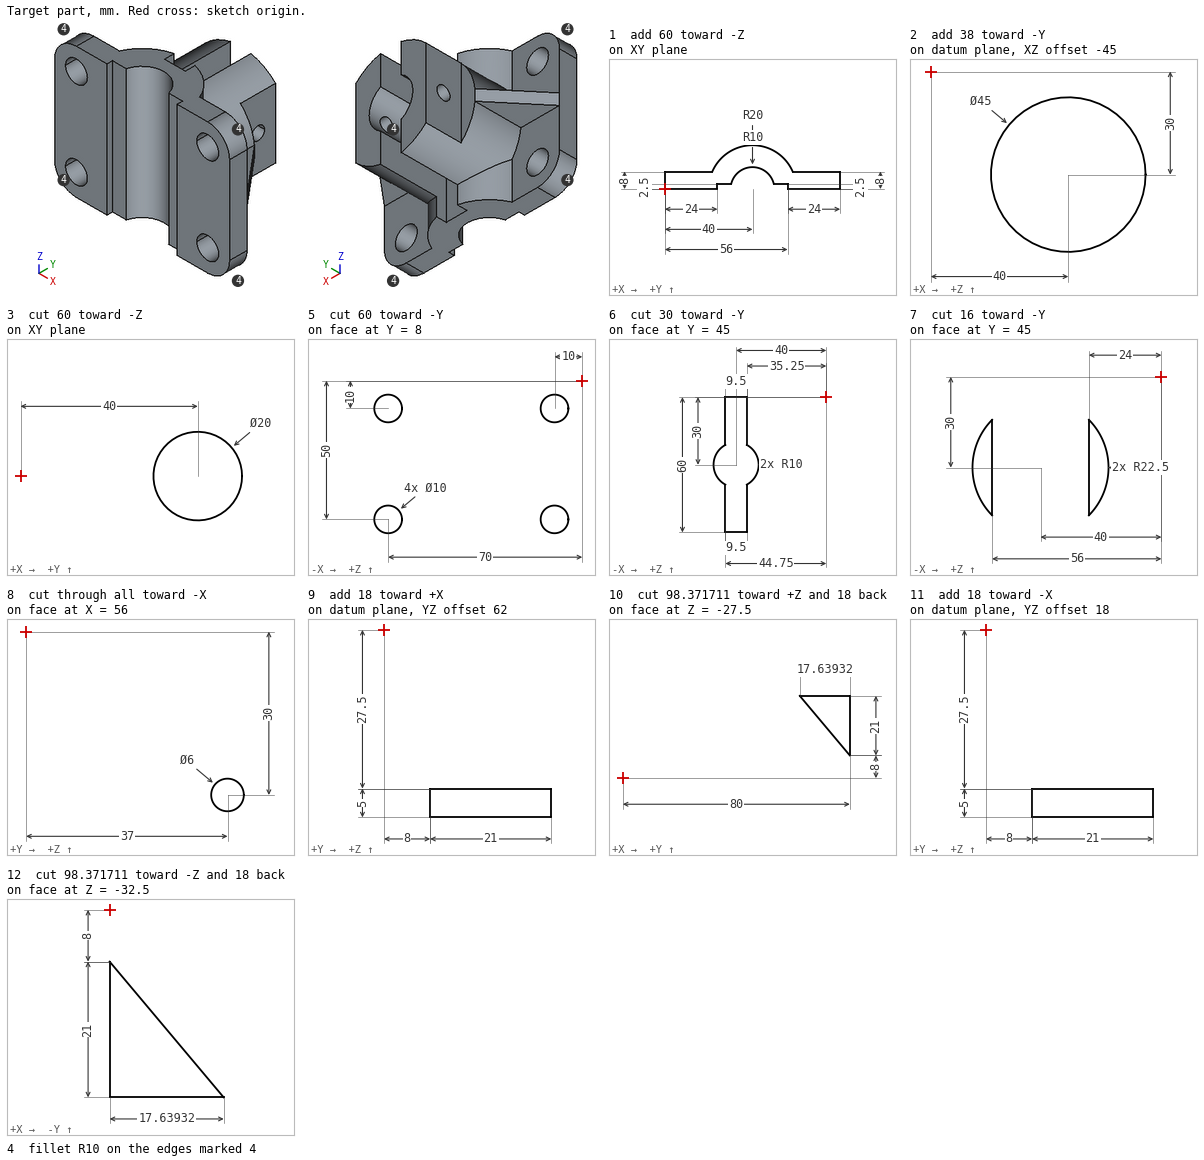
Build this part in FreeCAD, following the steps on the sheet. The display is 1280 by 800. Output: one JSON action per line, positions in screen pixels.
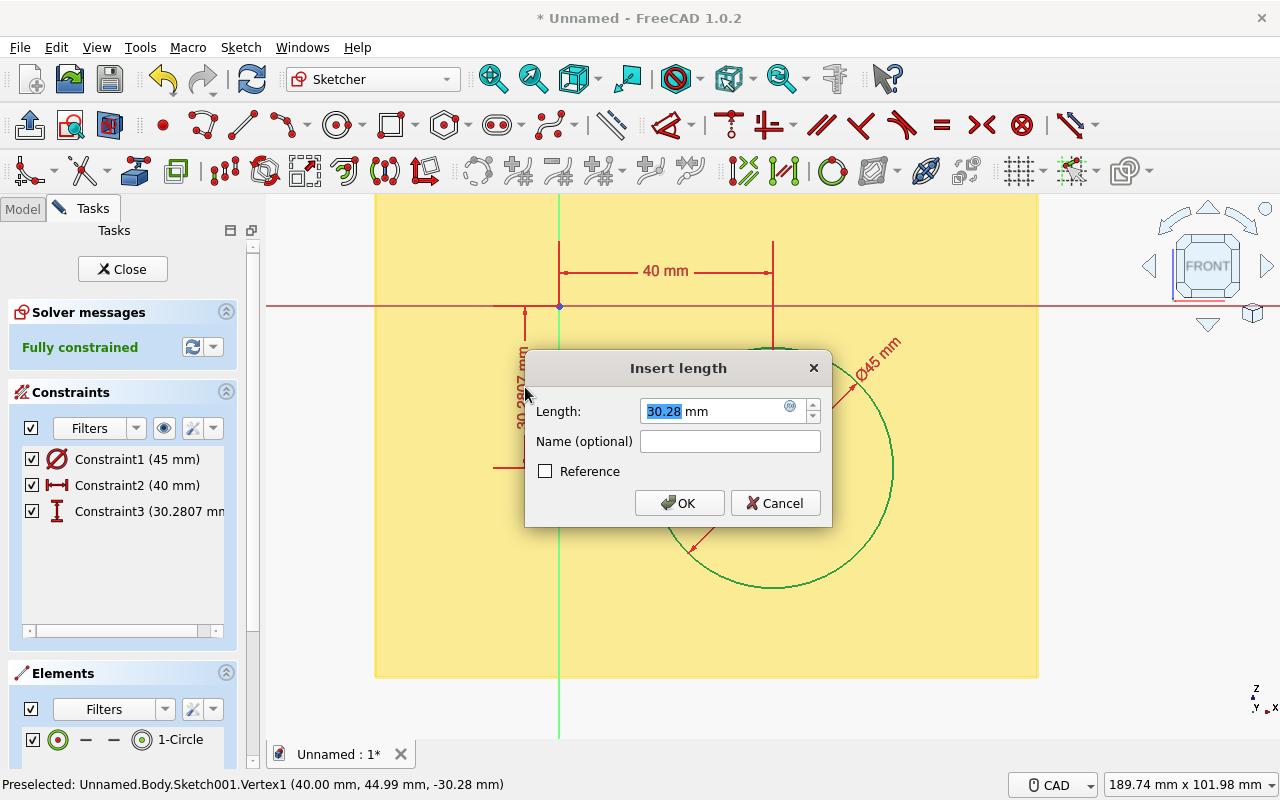
{"action": "type", "text": "30"}
{"action": "key", "text": "Return"}
{"action": "key", "text": "Escape"}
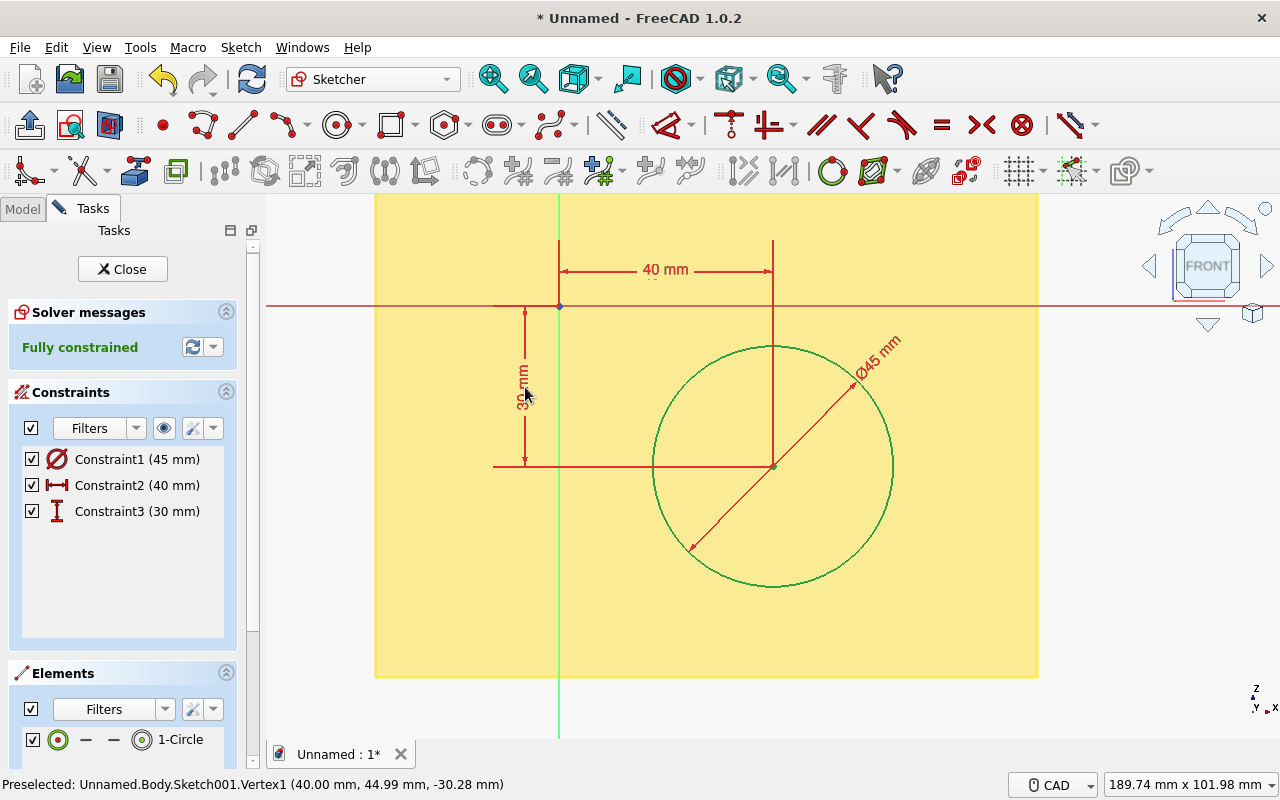
{"action": "left_click", "coordinate": [123, 269]}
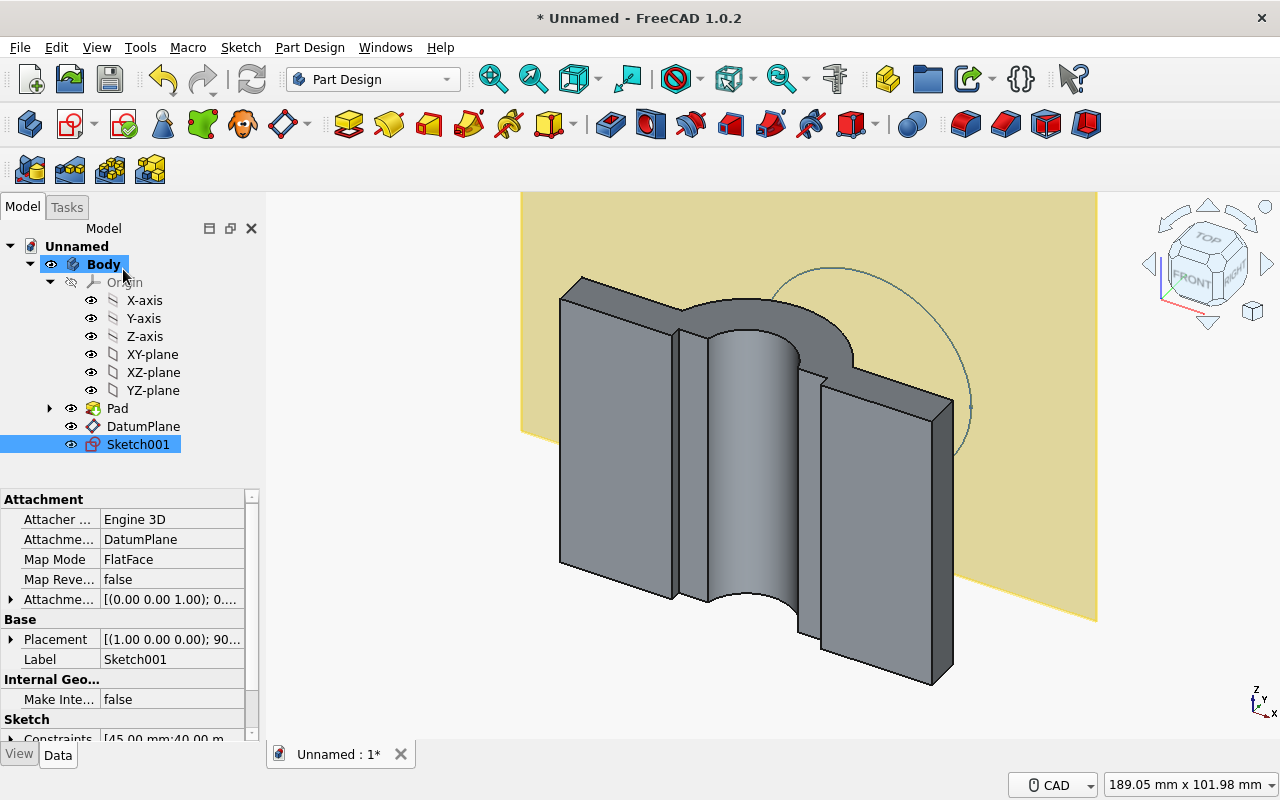
{"action": "left_click", "coordinate": [350, 124]}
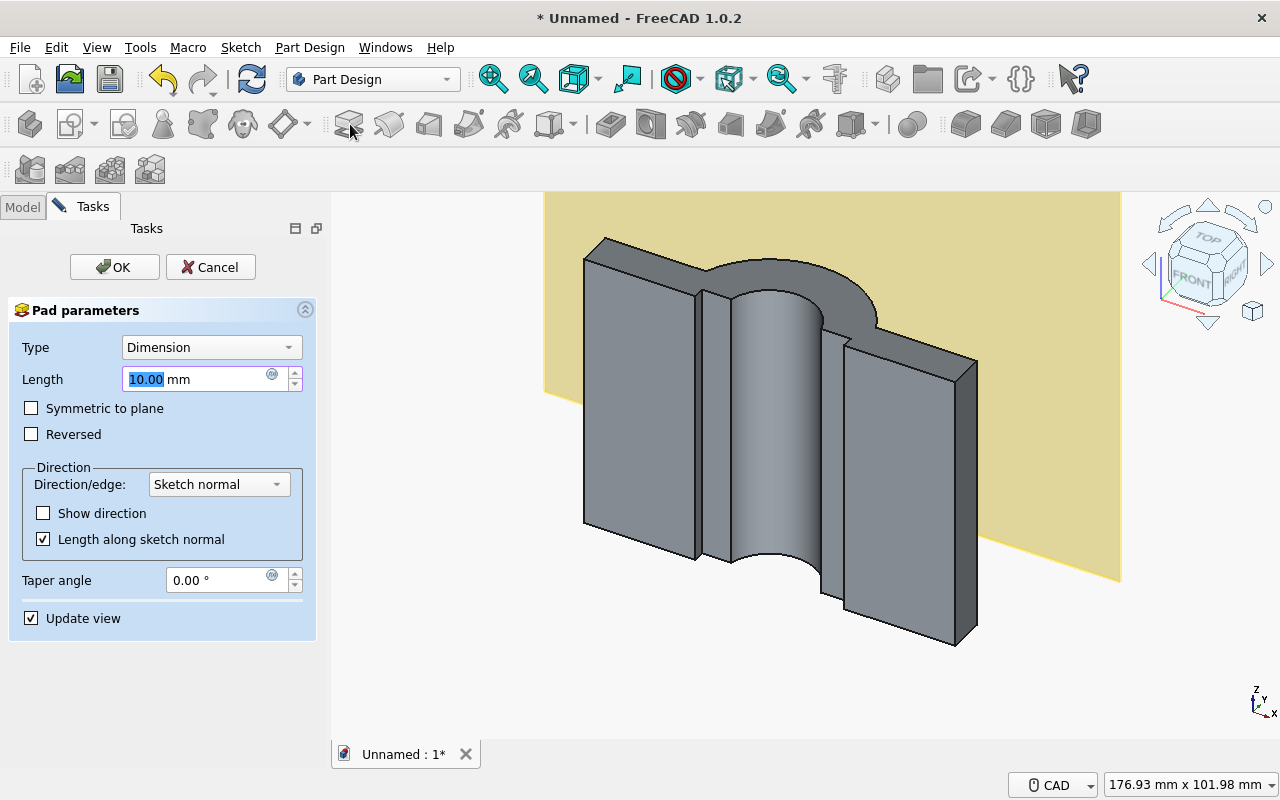
{"action": "type", "text": "38"}
{"action": "key", "text": "Tab"}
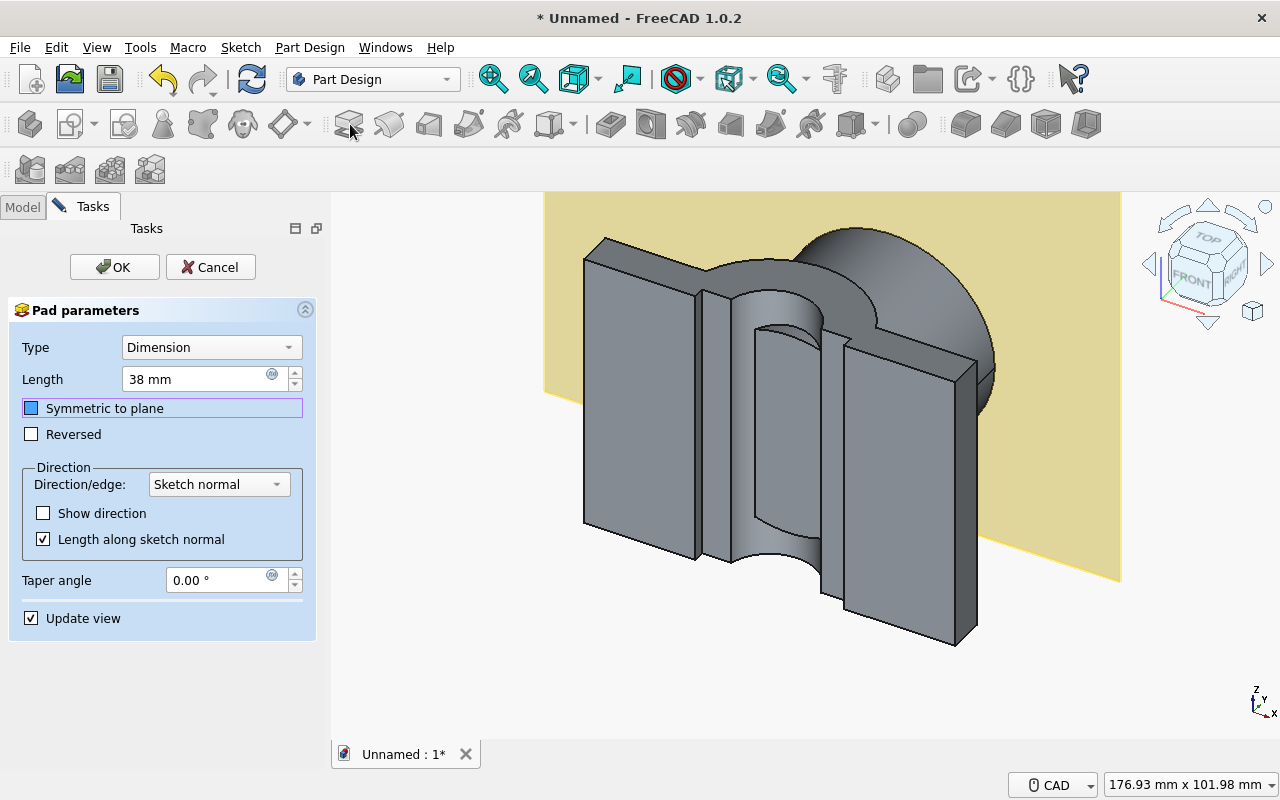
{"action": "left_click", "coordinate": [115, 267]}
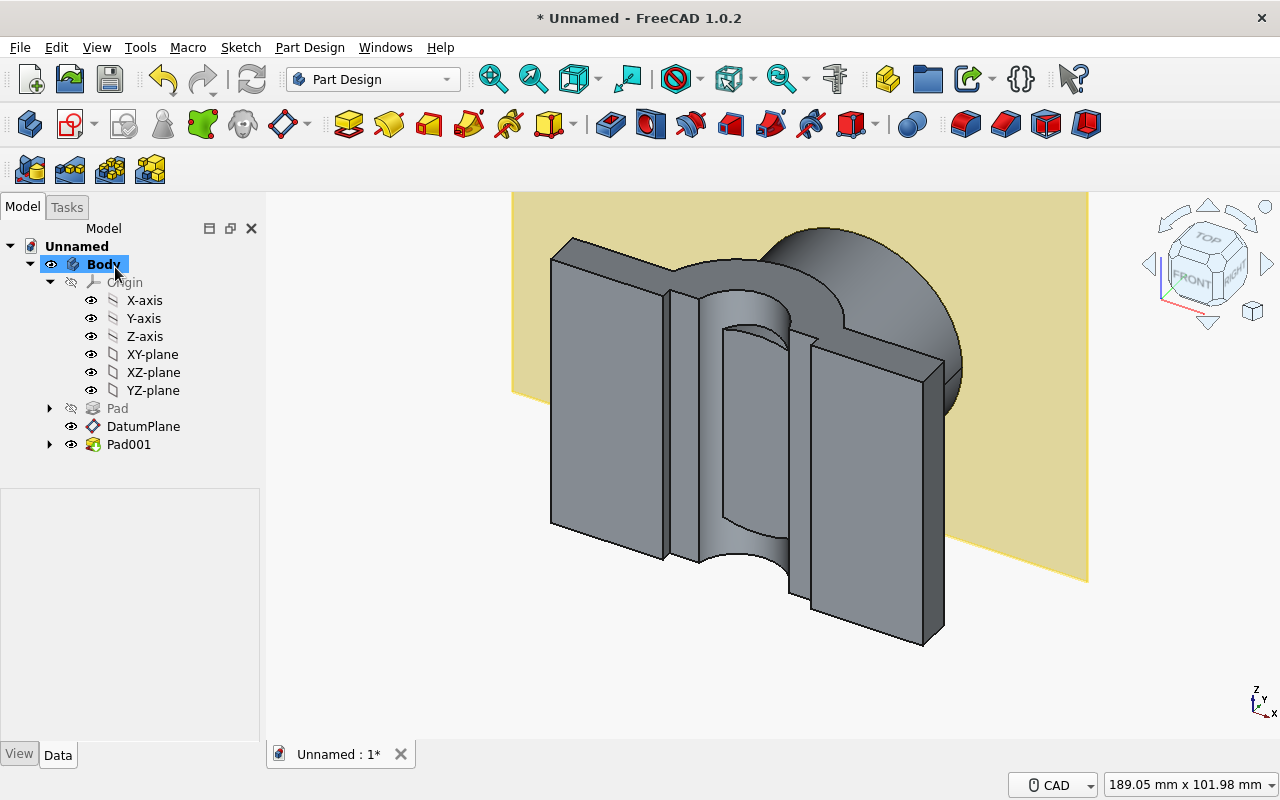
{"action": "left_click", "coordinate": [116, 426]}
{"action": "key", "text": "space"}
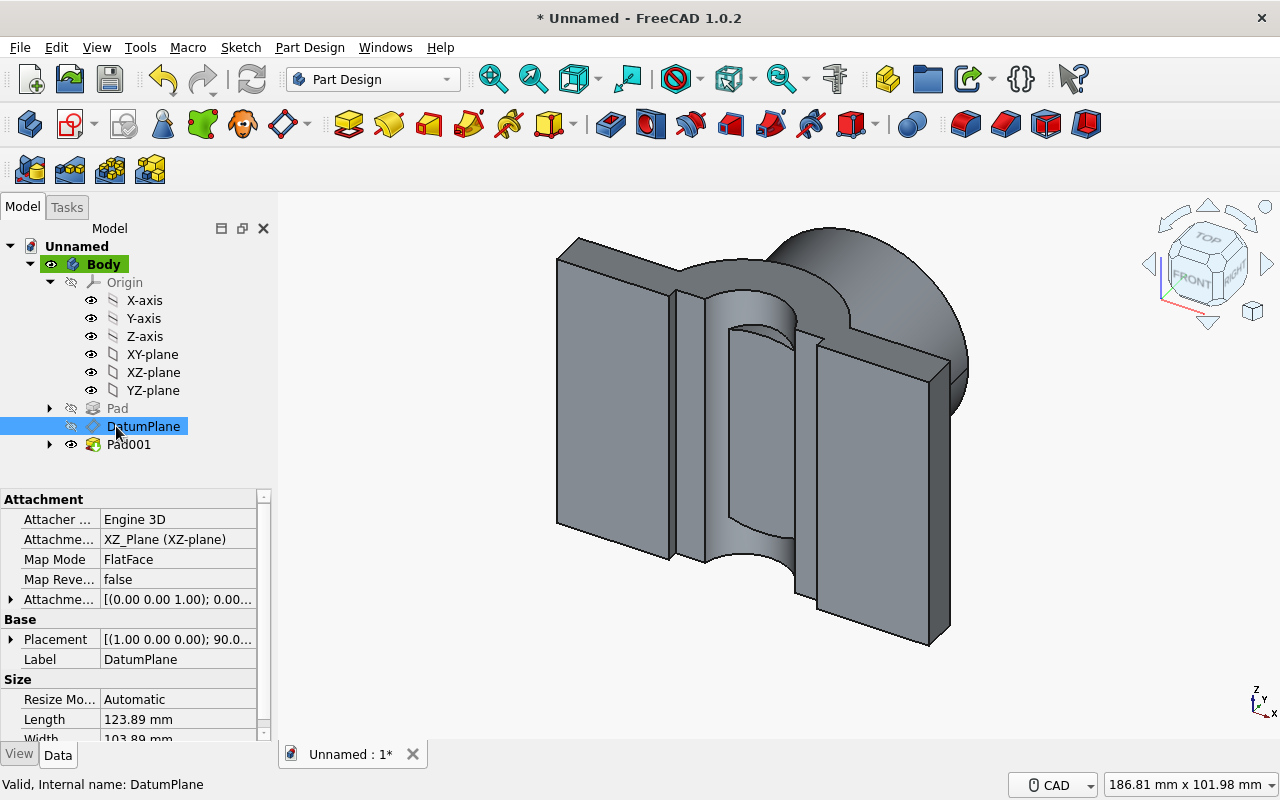
{"action": "left_click", "coordinate": [494, 80]}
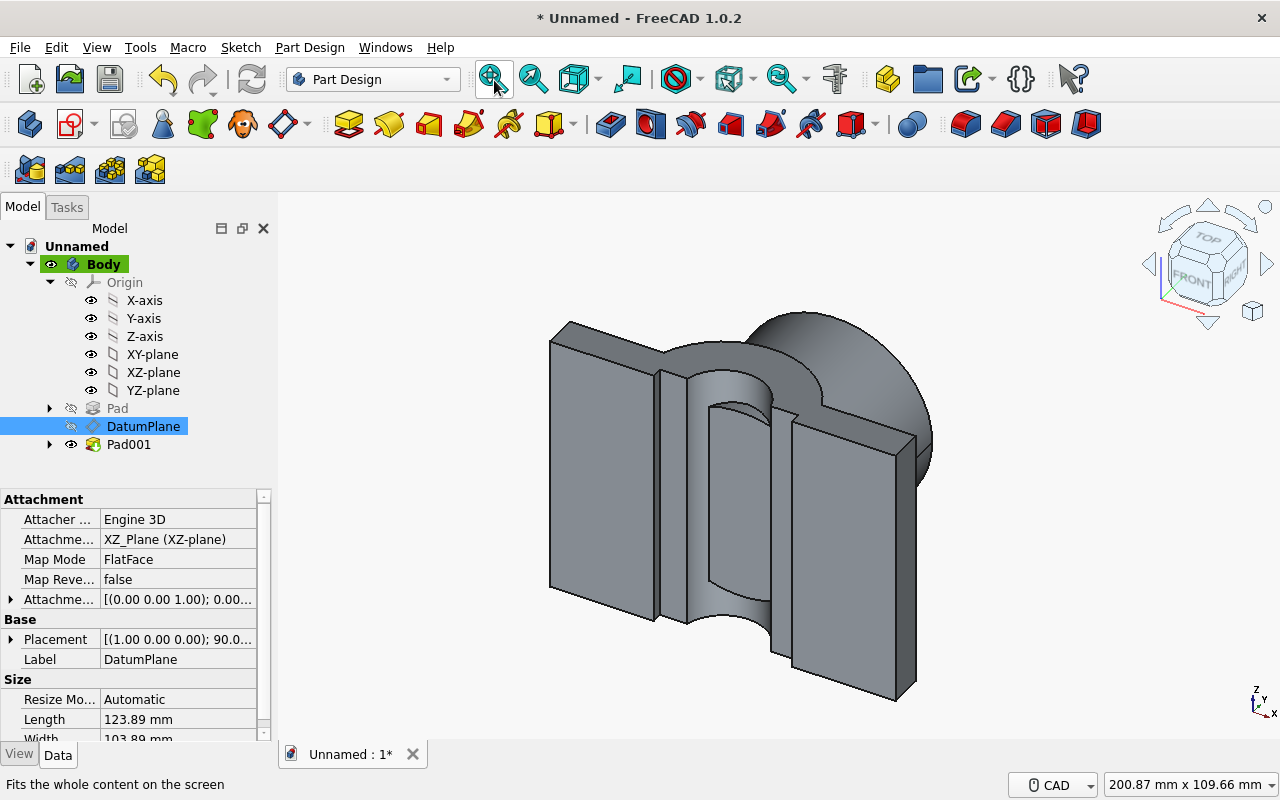
{"action": "left_click", "coordinate": [318, 699]}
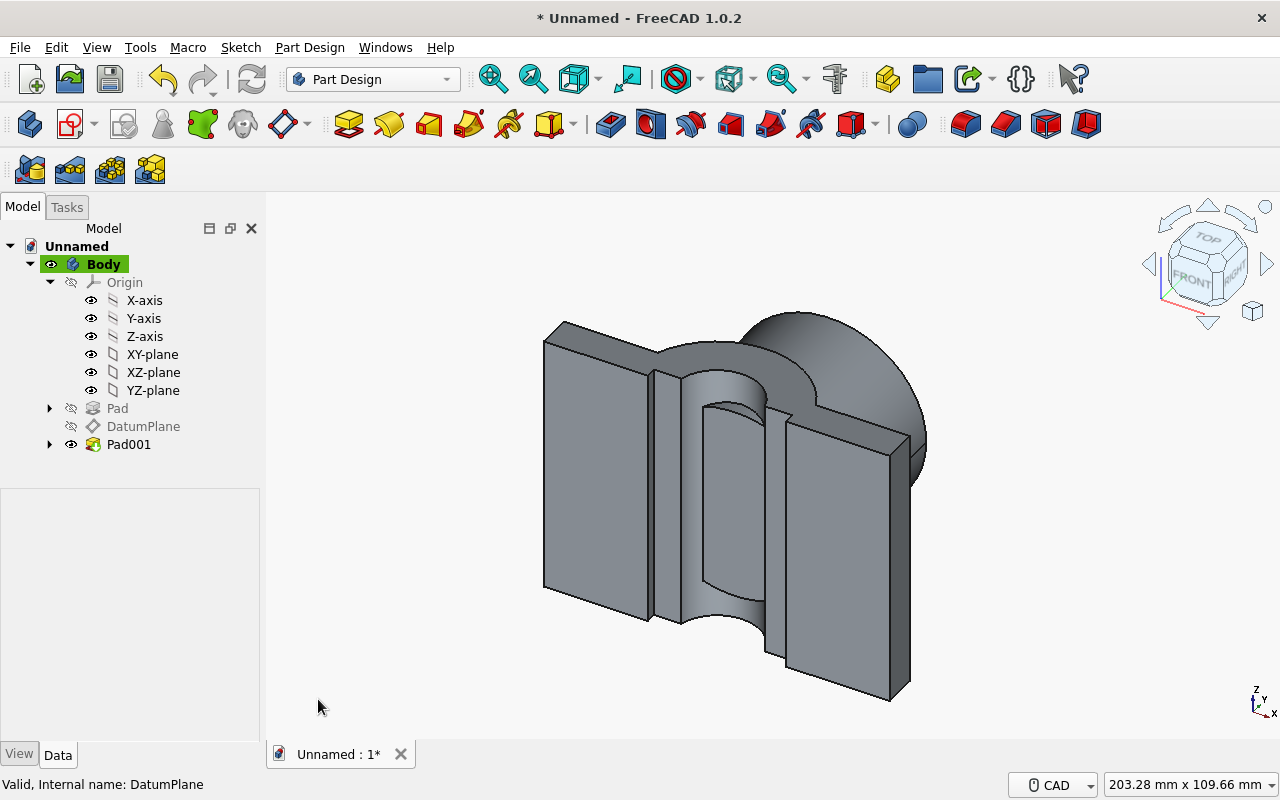
{"action": "left_click", "coordinate": [70, 124]}